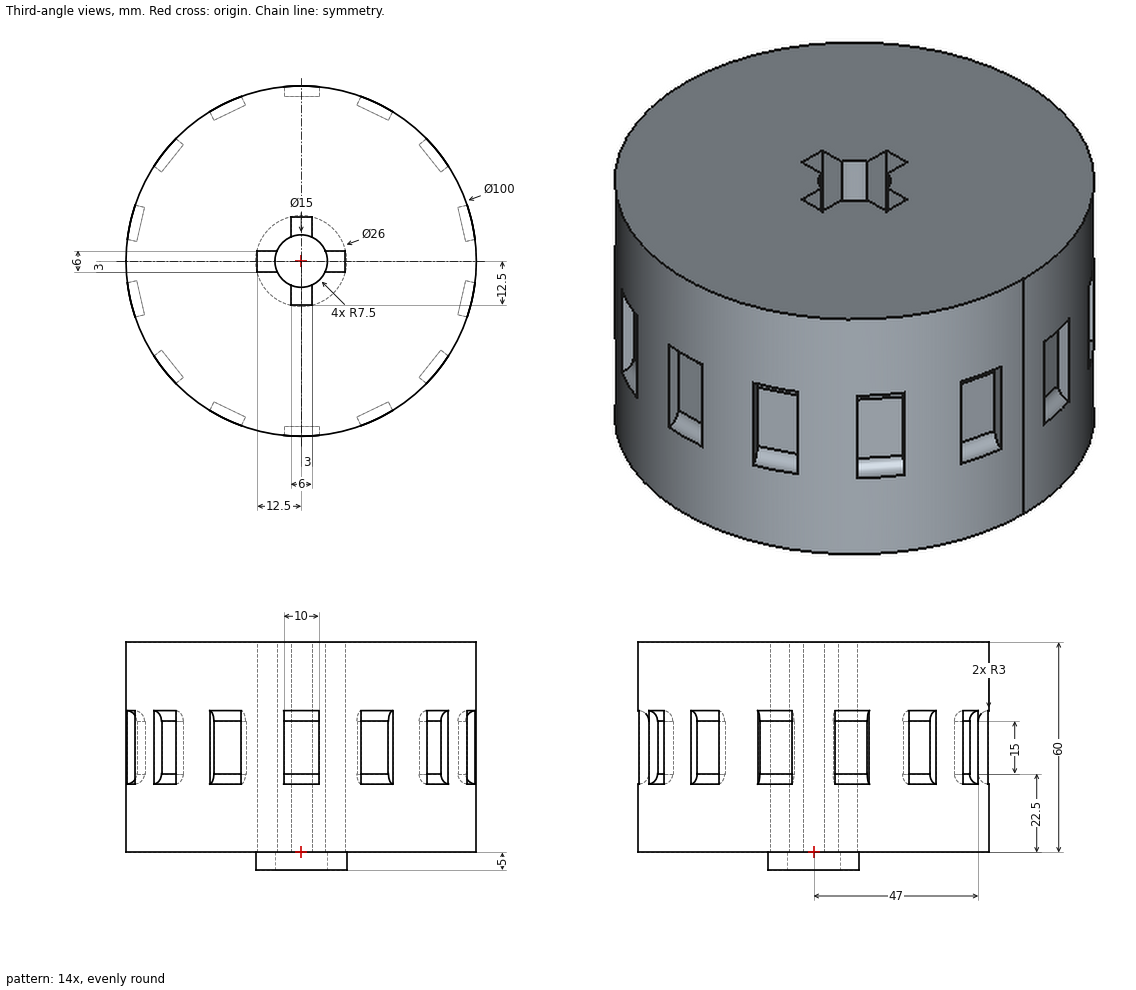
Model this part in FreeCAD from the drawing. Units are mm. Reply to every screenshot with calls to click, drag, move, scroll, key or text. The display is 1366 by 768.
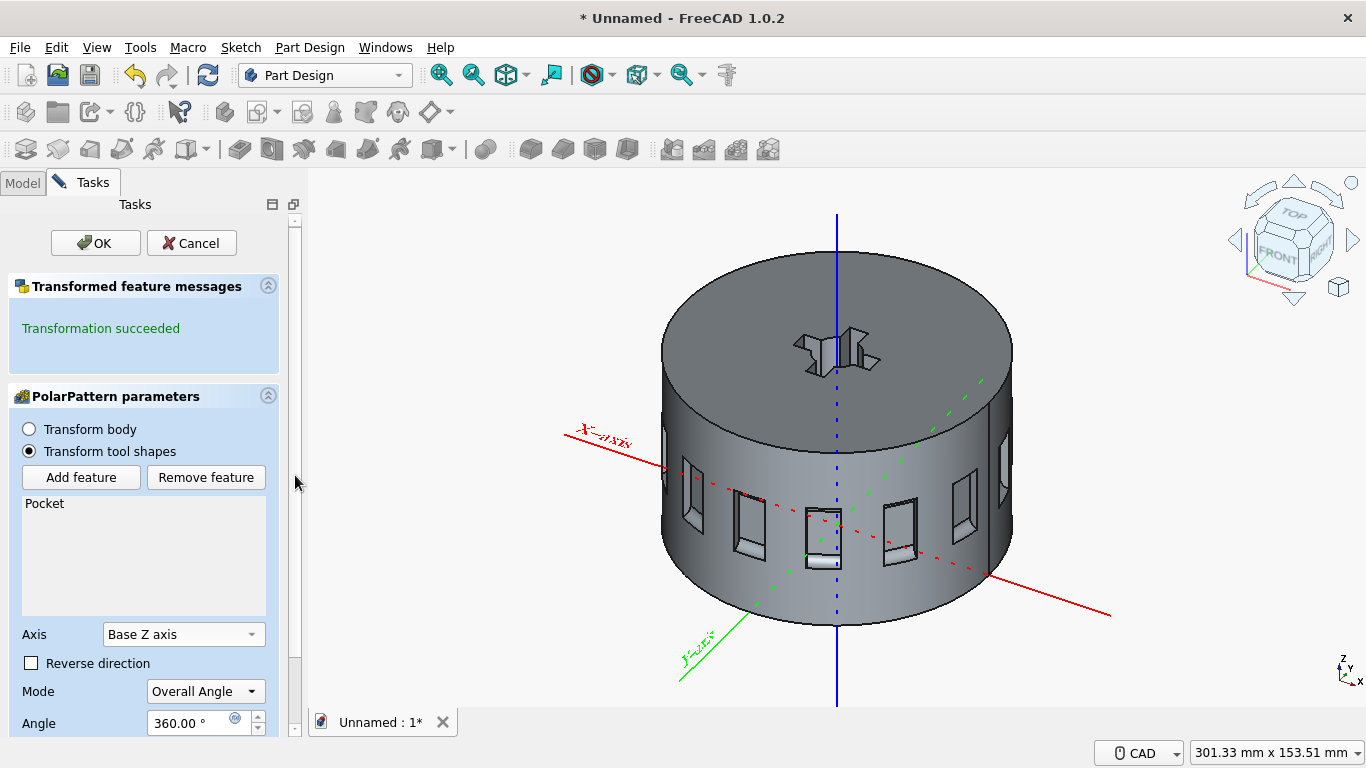
click(96, 243)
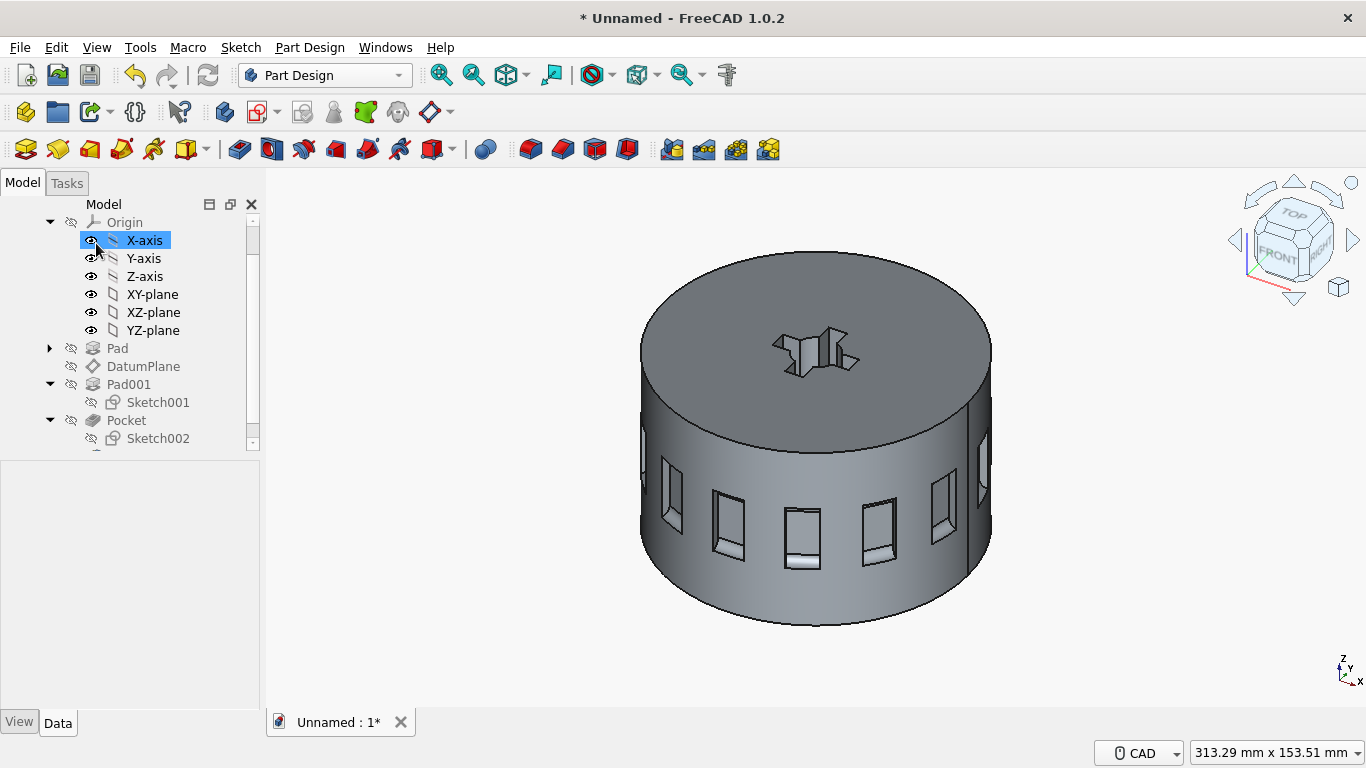
key(0)